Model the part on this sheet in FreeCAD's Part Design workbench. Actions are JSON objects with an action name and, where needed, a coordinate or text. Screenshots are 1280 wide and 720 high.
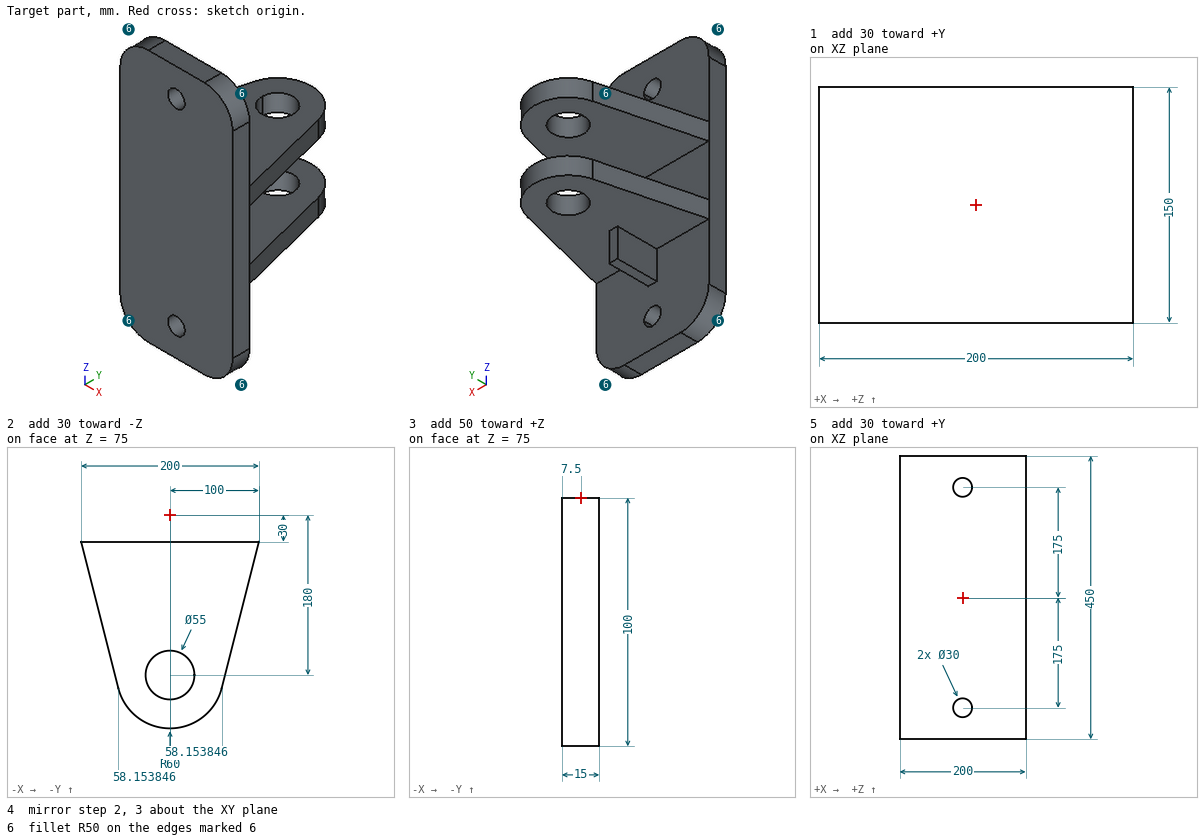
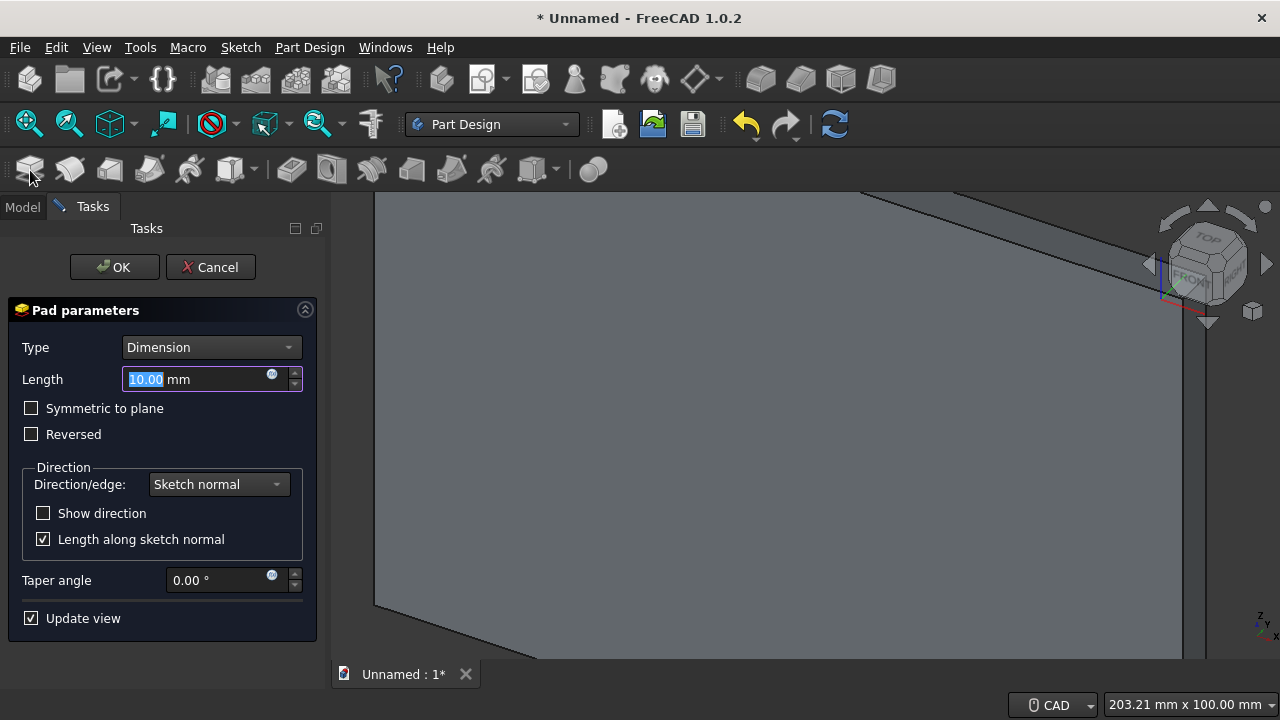
{"action": "type", "text": "30"}
{"action": "key", "text": "Tab"}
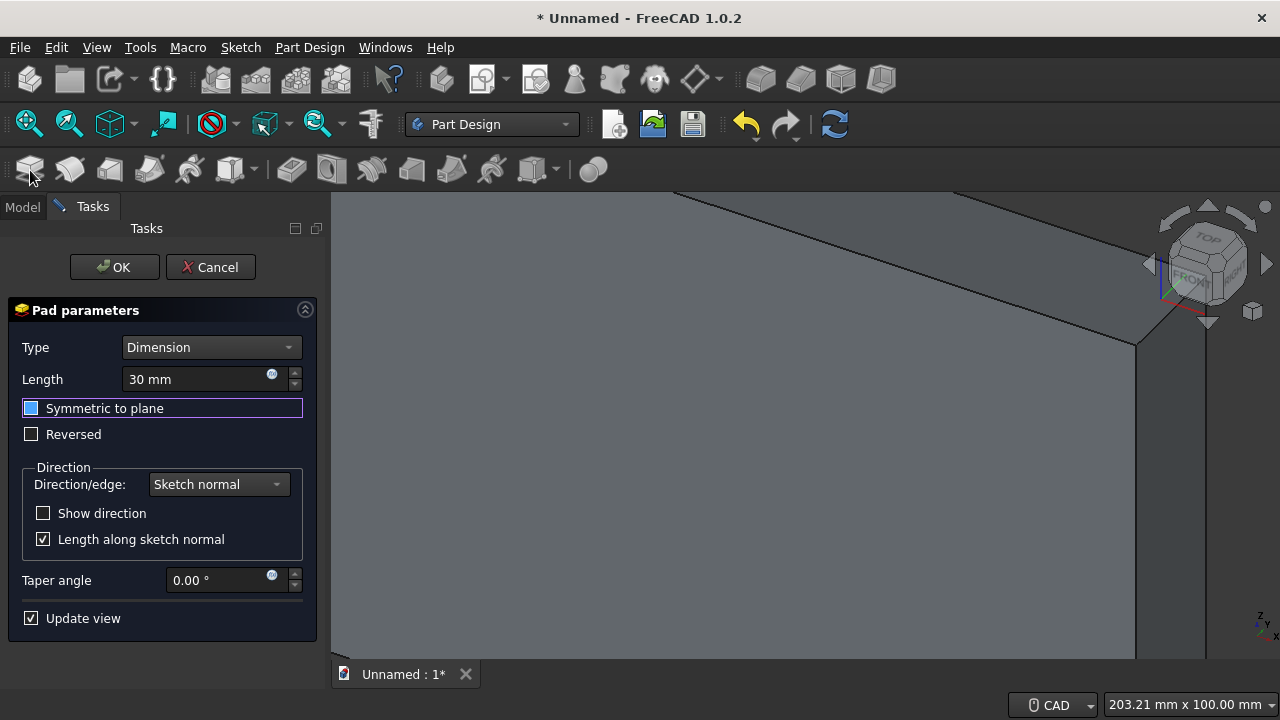
{"action": "left_click", "coordinate": [30, 434]}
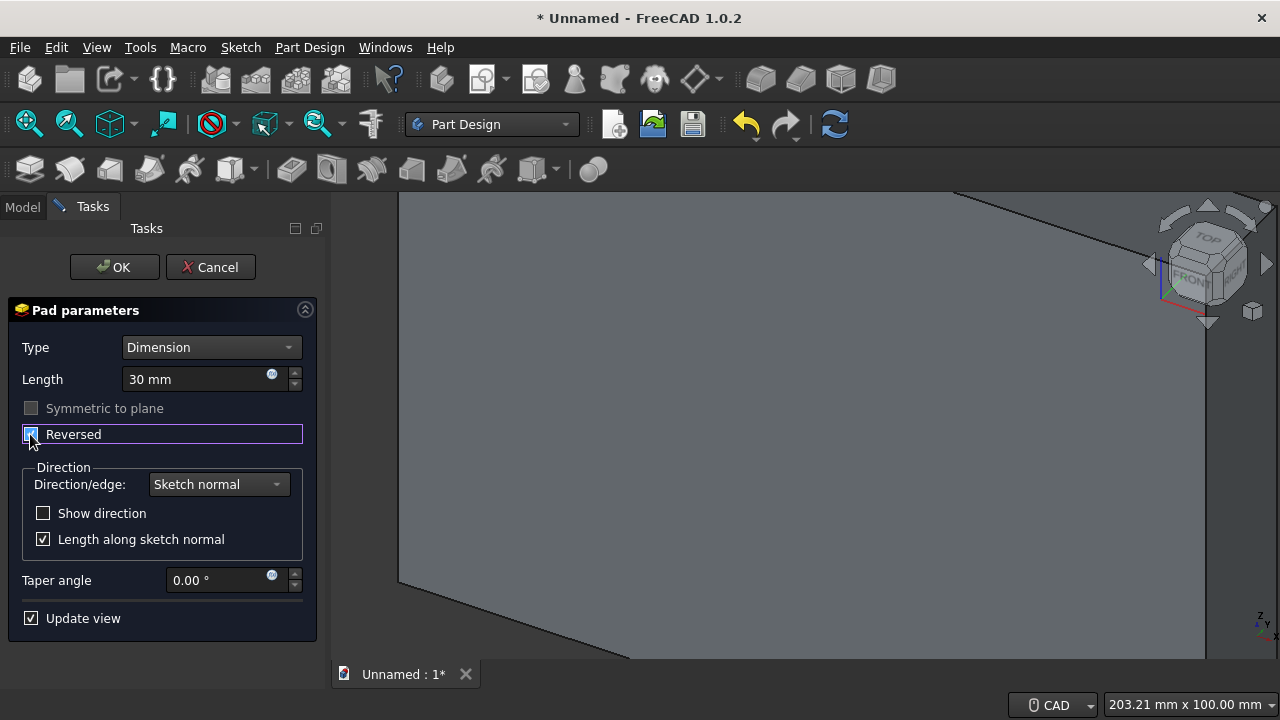
{"action": "left_click", "coordinate": [115, 267]}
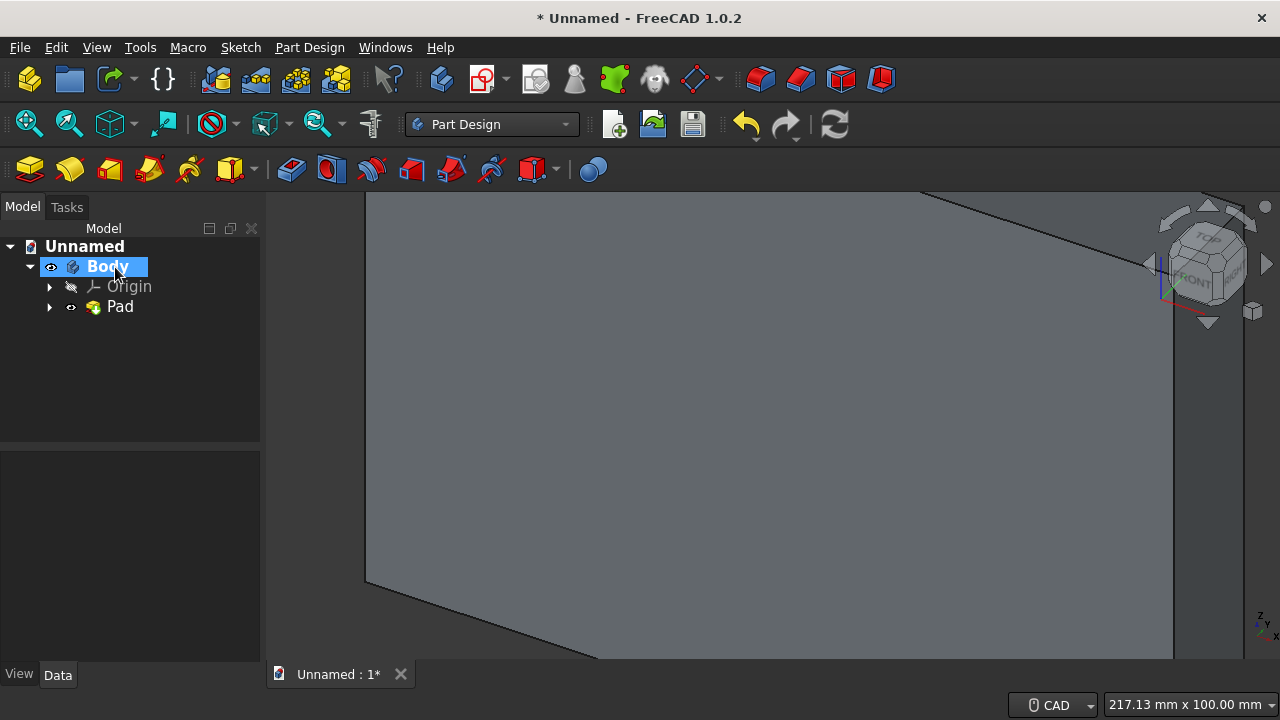
{"action": "key", "text": "v f"}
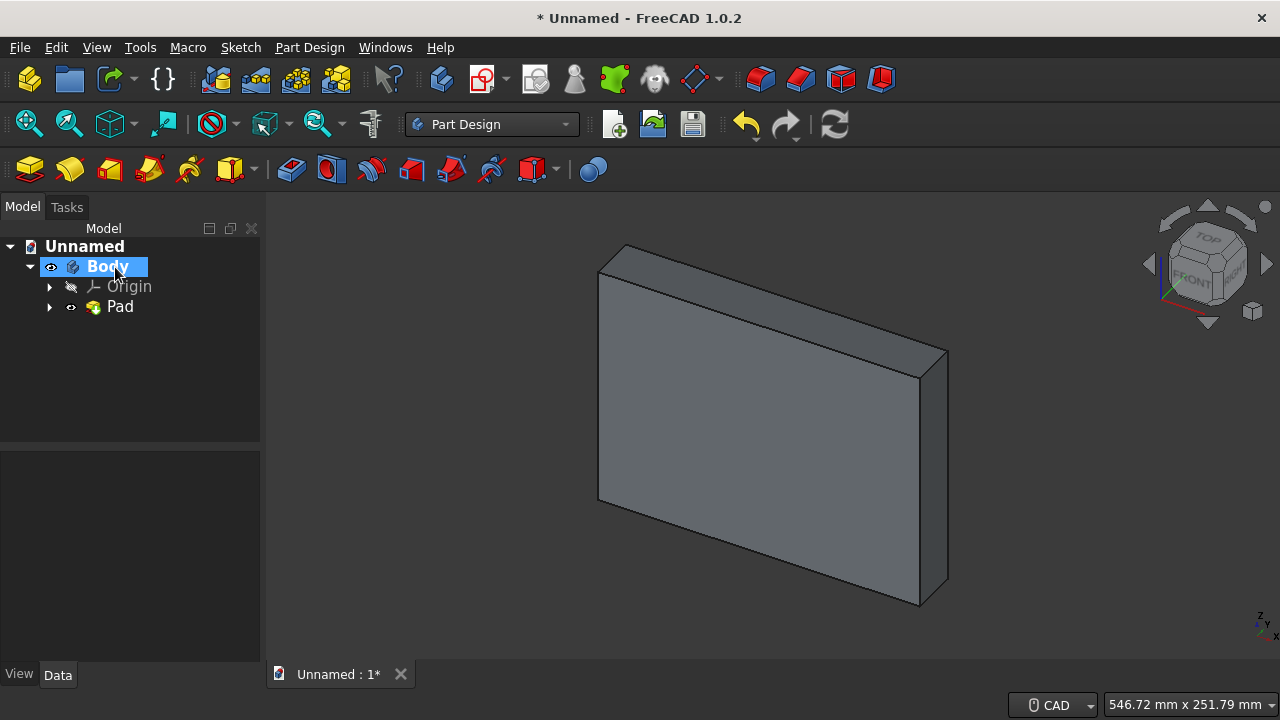
{"action": "left_click", "coordinate": [865, 341]}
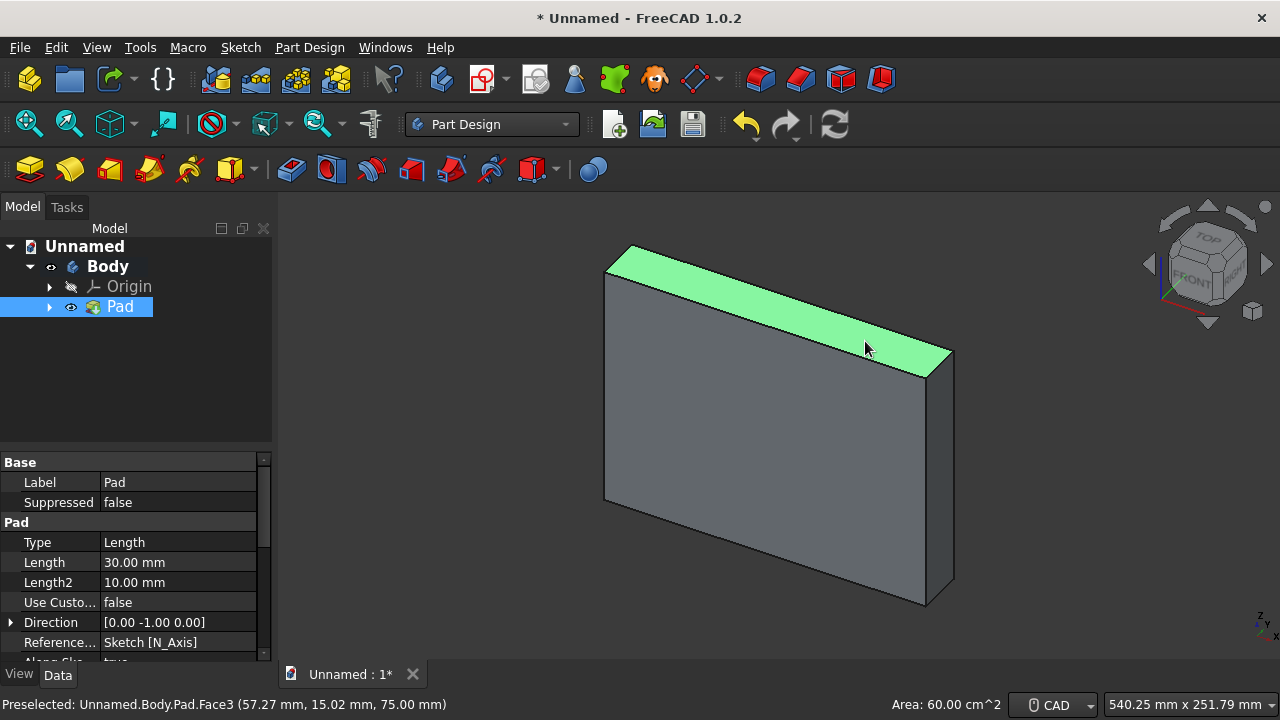
{"action": "left_click", "coordinate": [482, 80]}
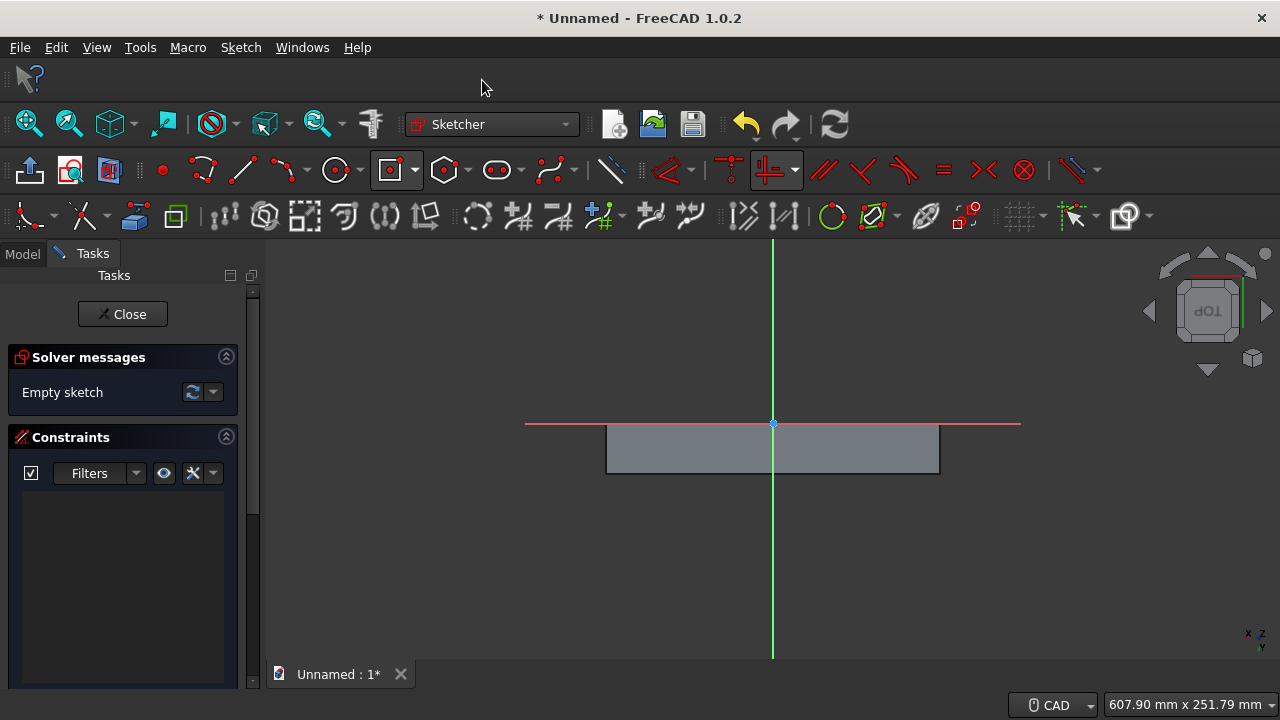
{"action": "scroll", "coordinate": [621, 267], "scroll_direction": "down", "scroll_amount": 3}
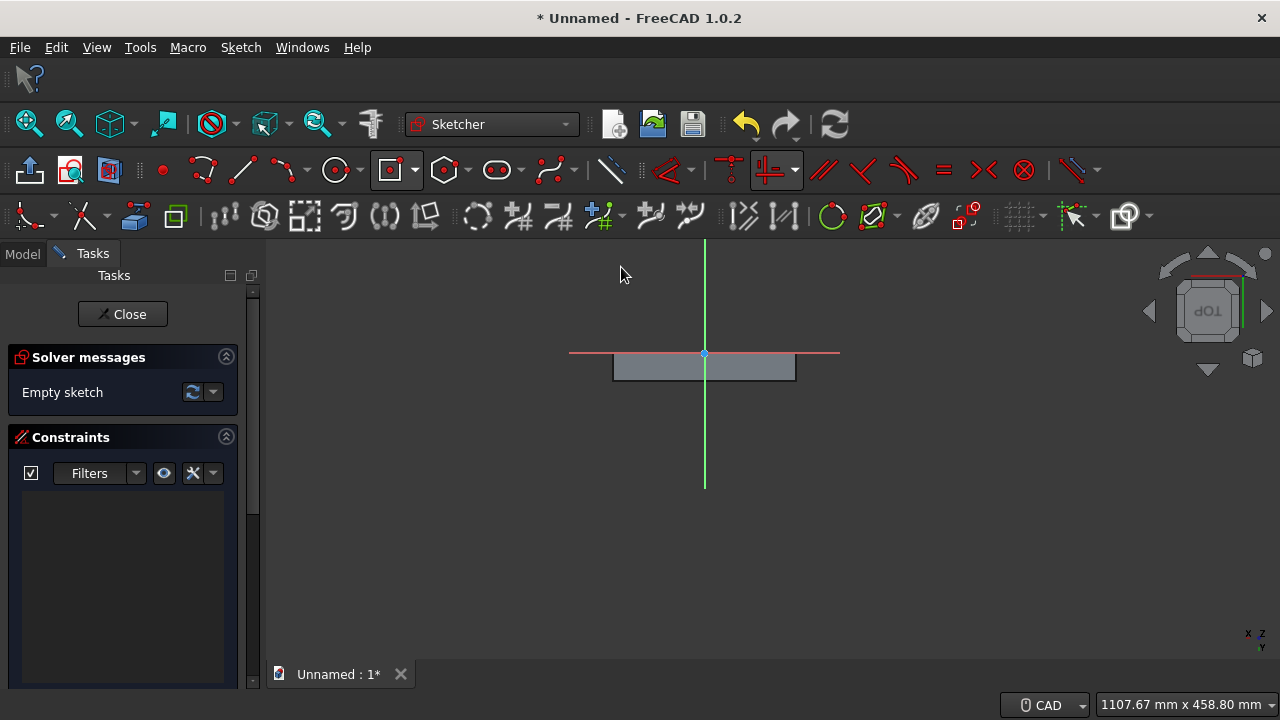
{"action": "key", "text": "g m"}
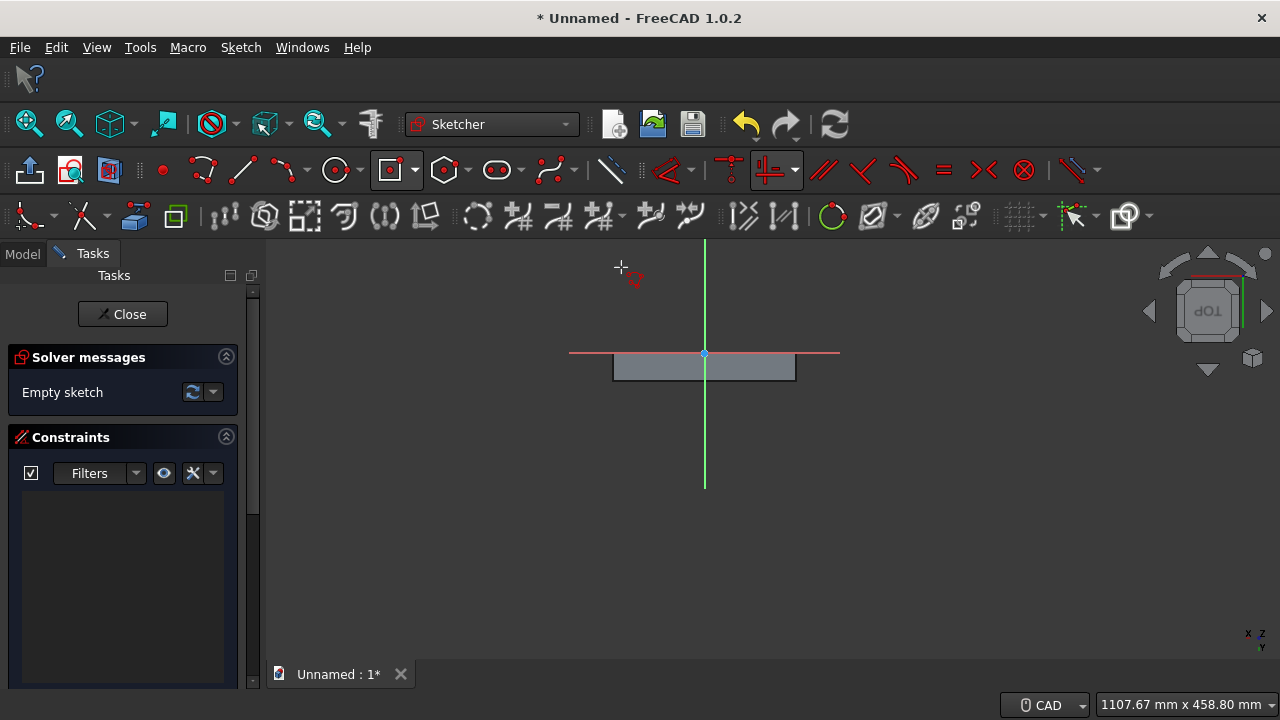
{"action": "left_click", "coordinate": [758, 531]}
{"action": "left_click", "coordinate": [796, 381]}
{"action": "left_click", "coordinate": [613, 381]}
{"action": "left_click", "coordinate": [651, 531]}
{"action": "right_click", "coordinate": [651, 531]}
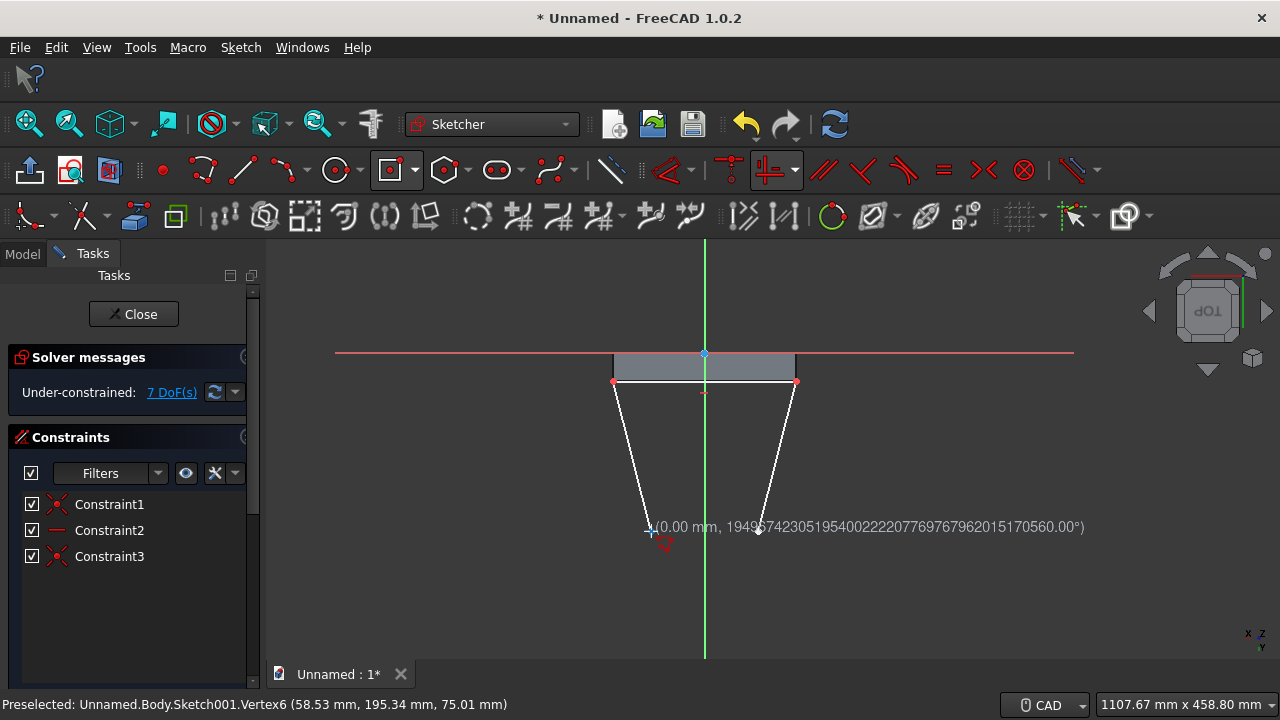
{"action": "left_click", "coordinate": [284, 170]}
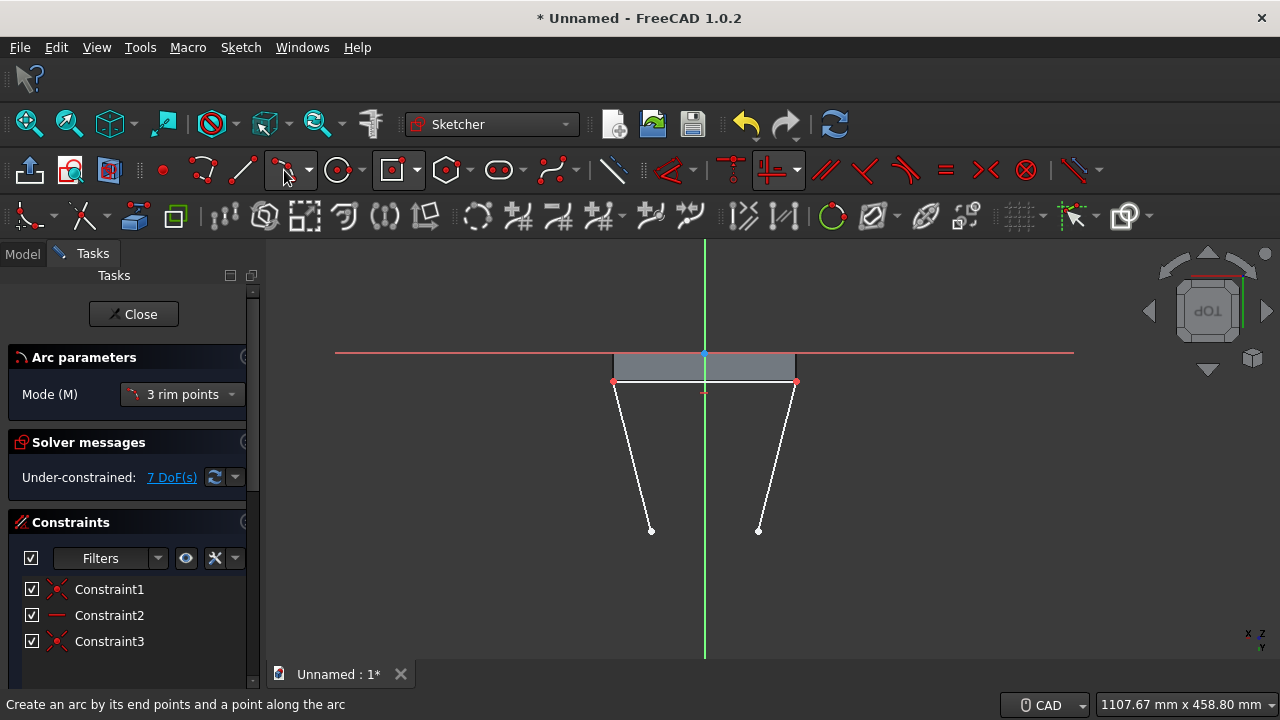
{"action": "left_click", "coordinate": [651, 532]}
{"action": "left_click", "coordinate": [758, 532]}
{"action": "left_click", "coordinate": [690, 571]}